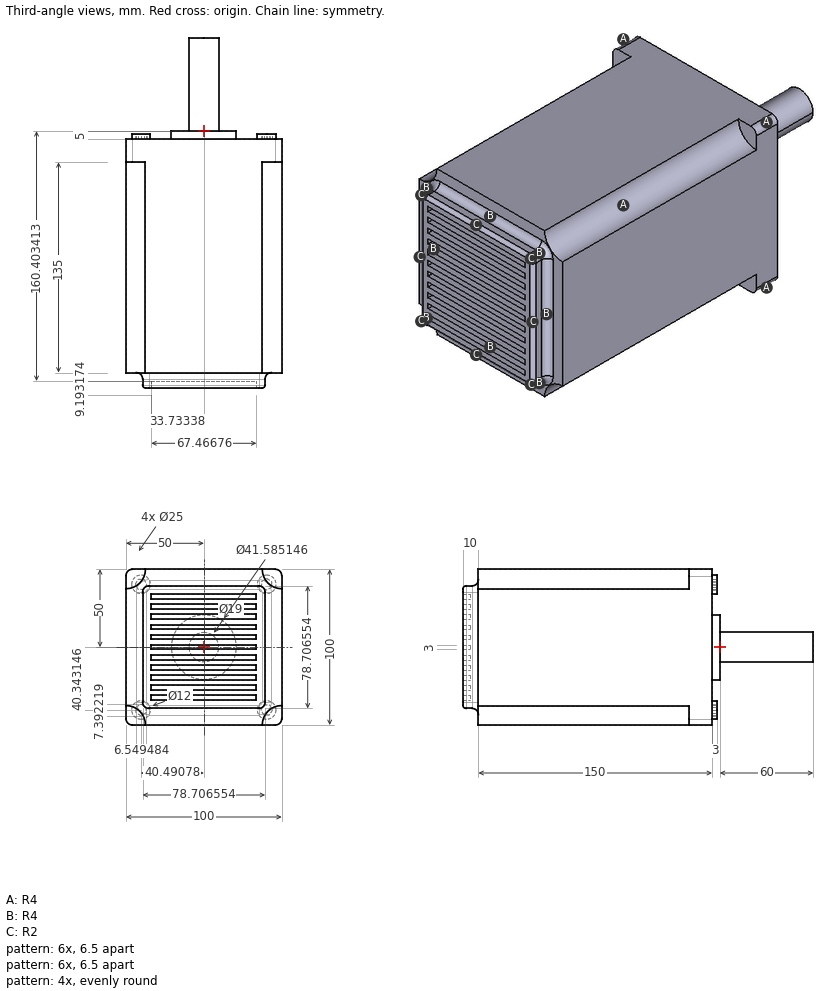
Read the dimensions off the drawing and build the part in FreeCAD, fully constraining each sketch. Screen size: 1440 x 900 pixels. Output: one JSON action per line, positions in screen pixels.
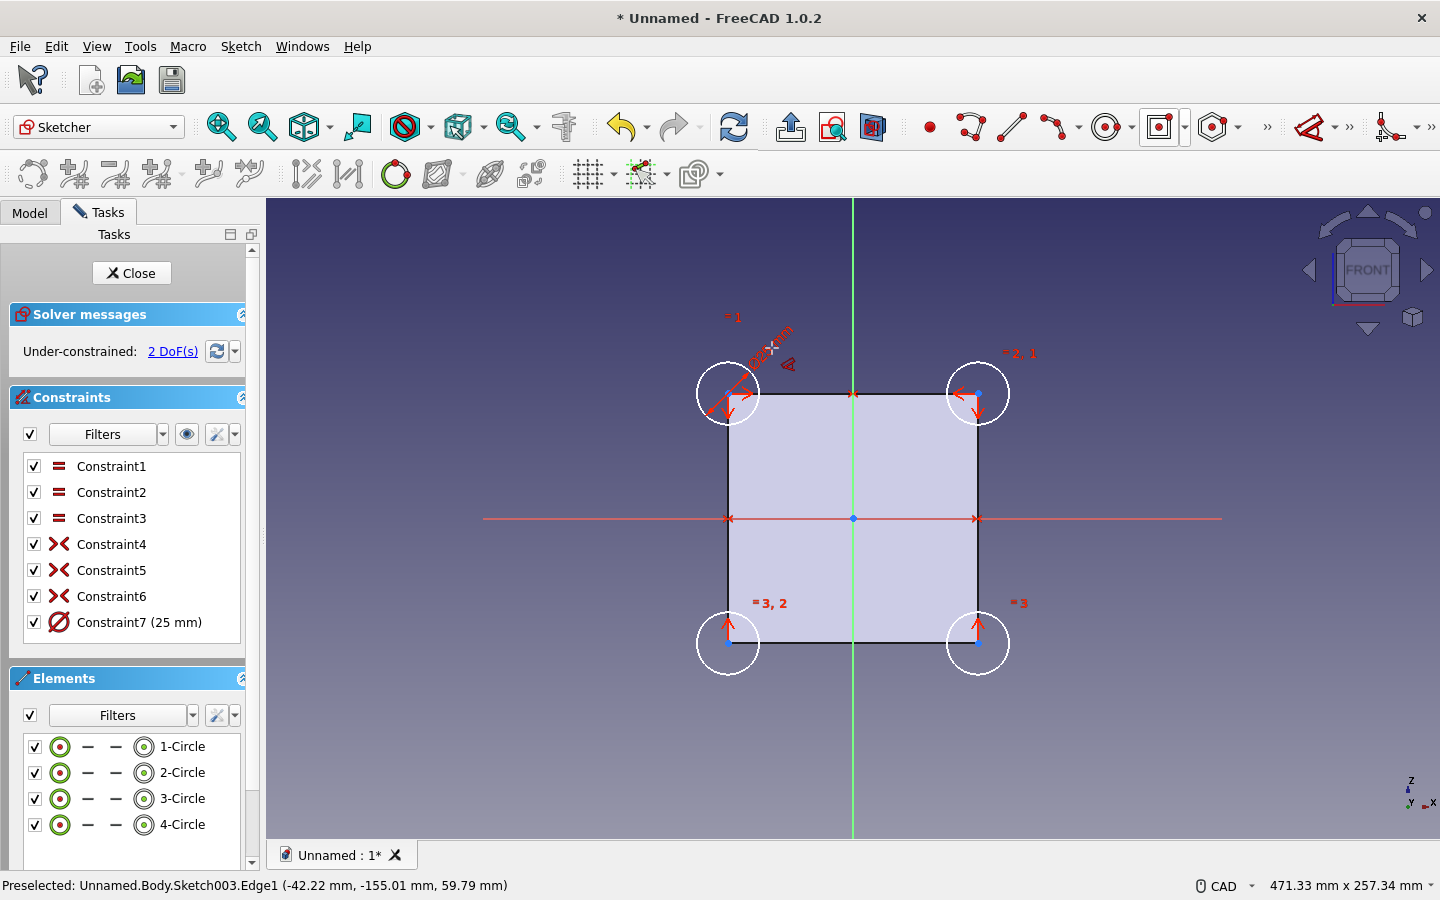
{"action": "left_click", "coordinate": [728, 394]}
{"action": "left_click", "coordinate": [791, 552]}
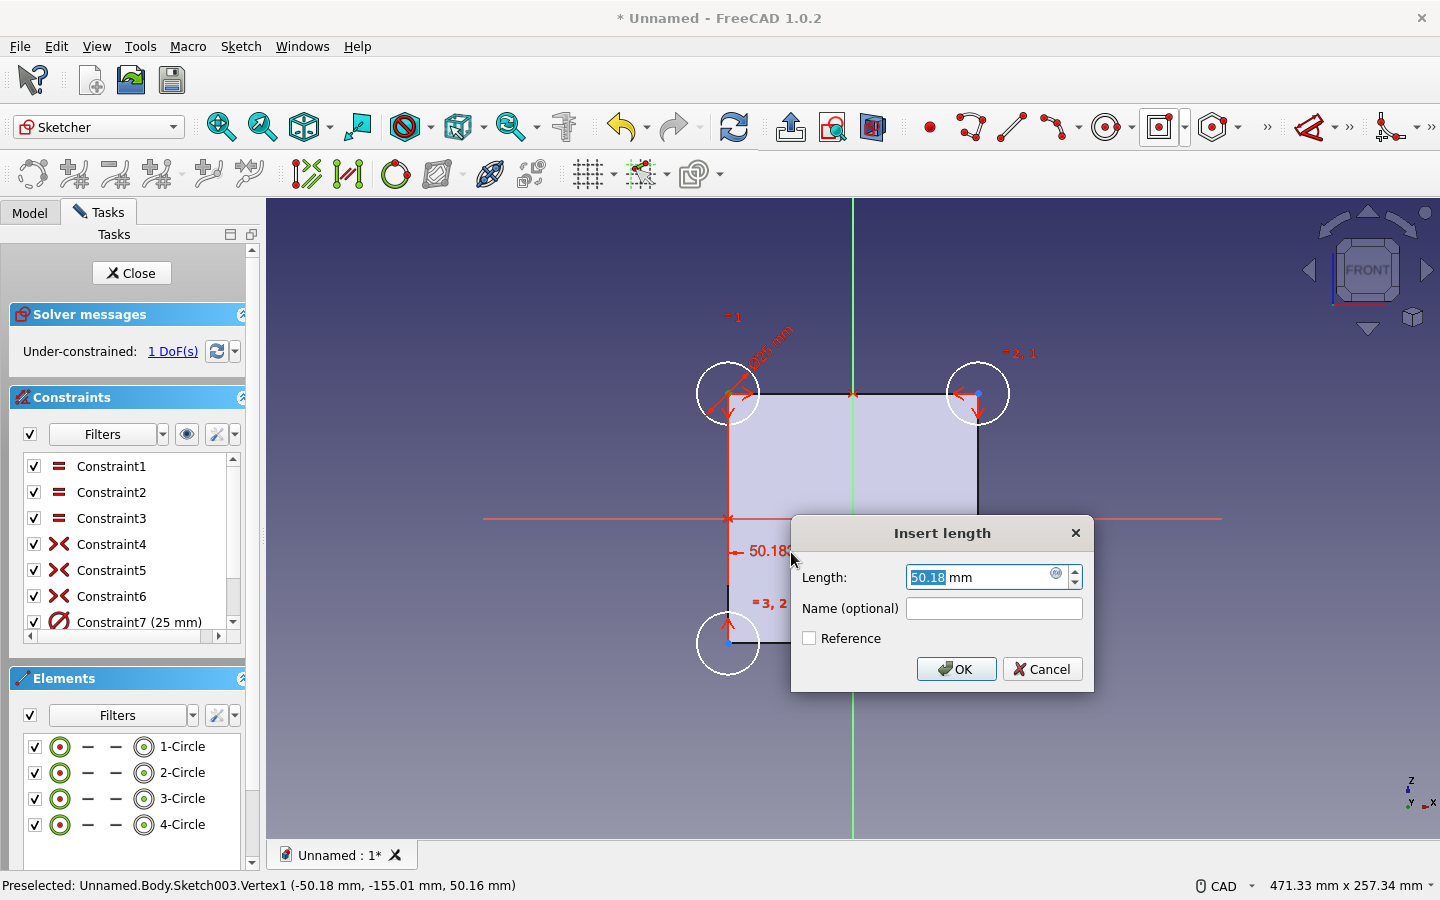
{"action": "type", "text": "50"}
{"action": "key", "text": "Return"}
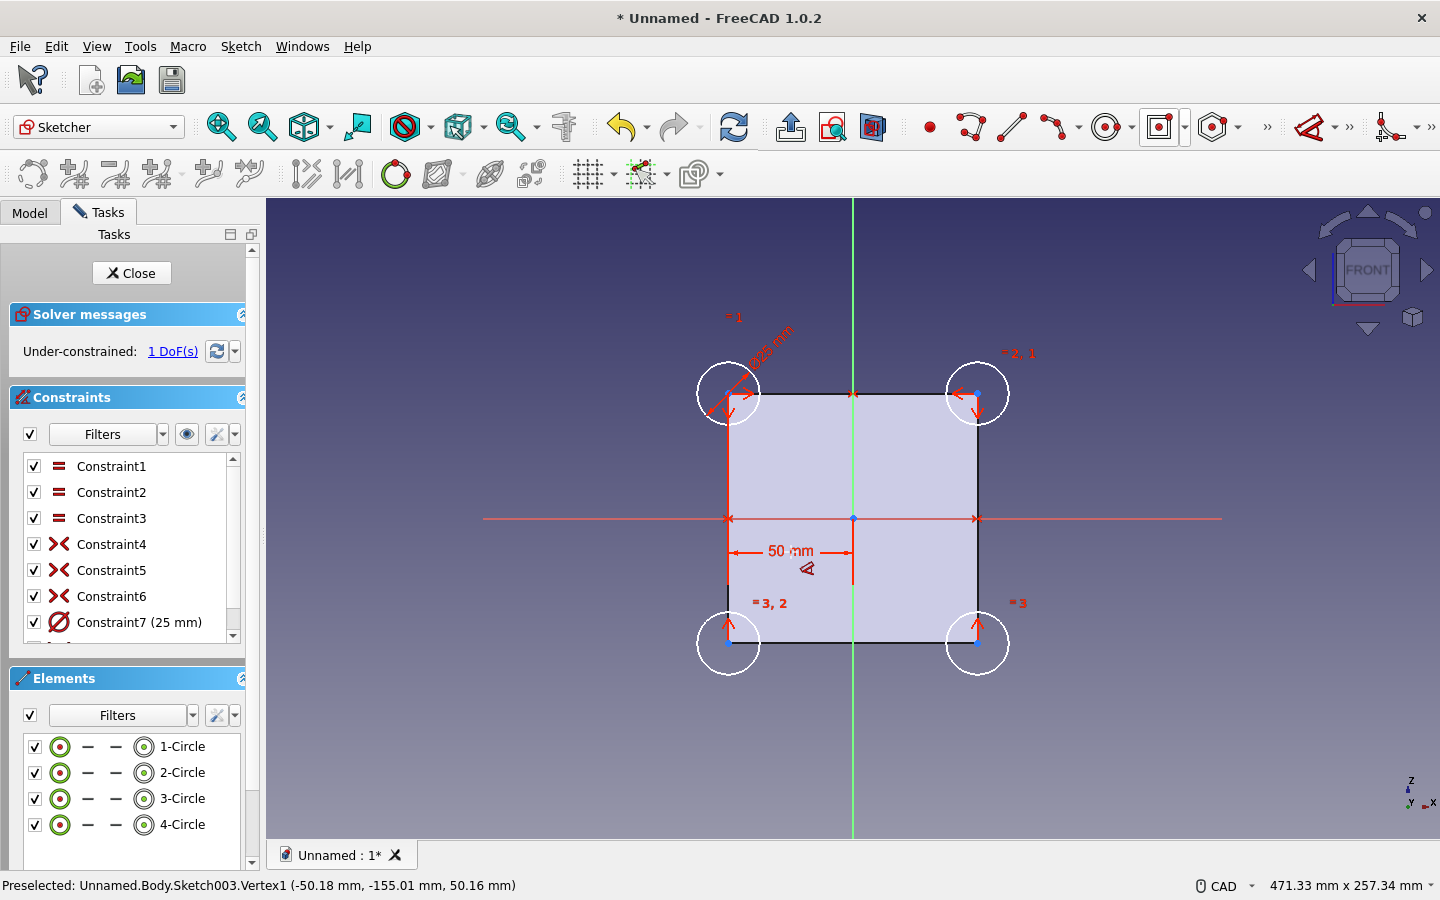
{"action": "left_click", "coordinate": [728, 394]}
{"action": "left_click", "coordinate": [694, 456]}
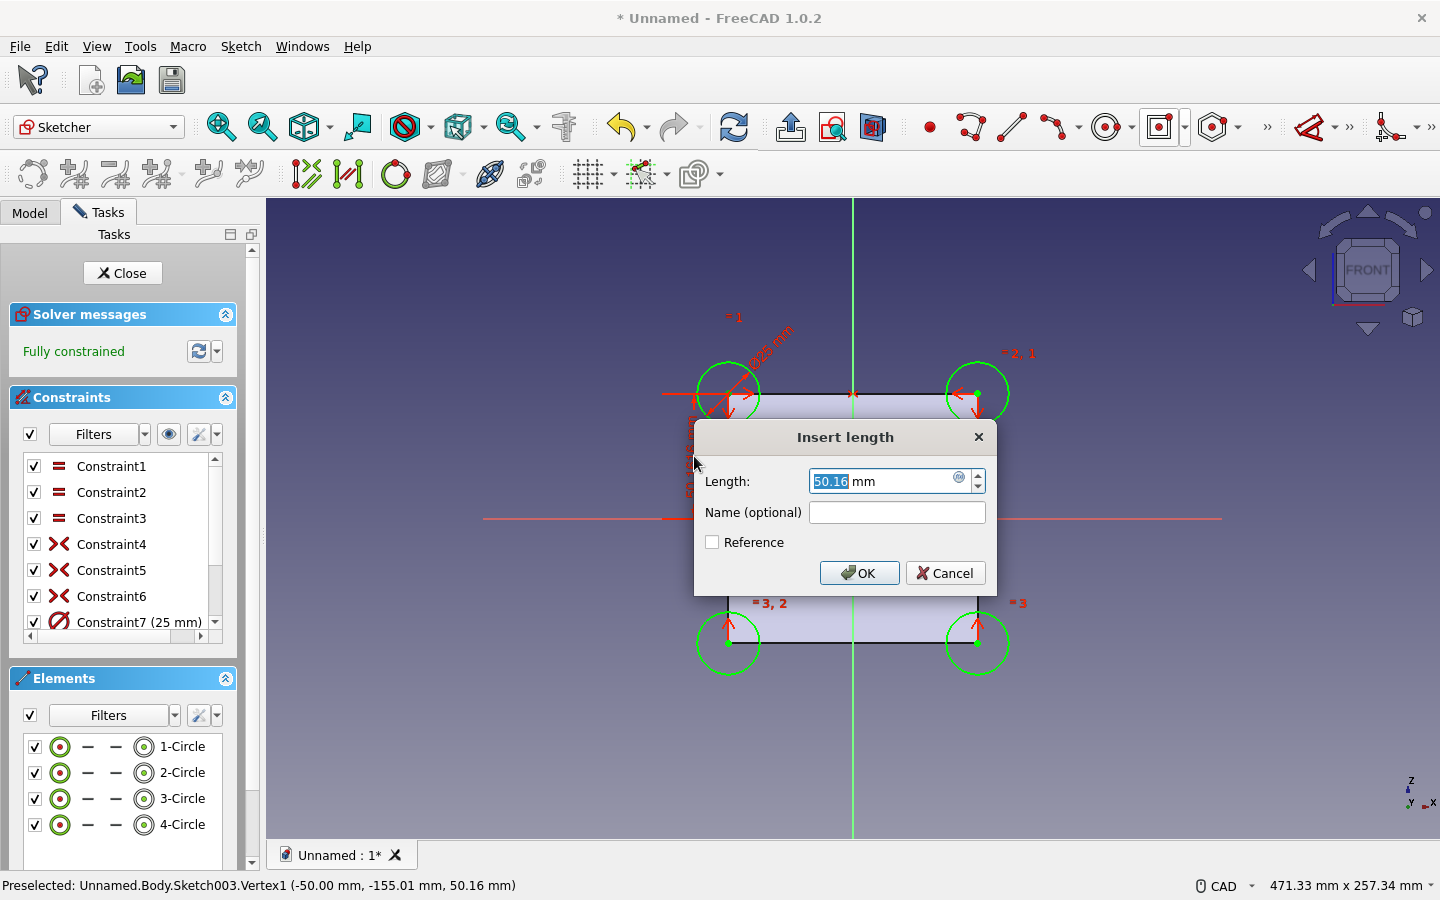
{"action": "type", "text": "50"}
{"action": "key", "text": "Return"}
{"action": "key", "text": "Escape"}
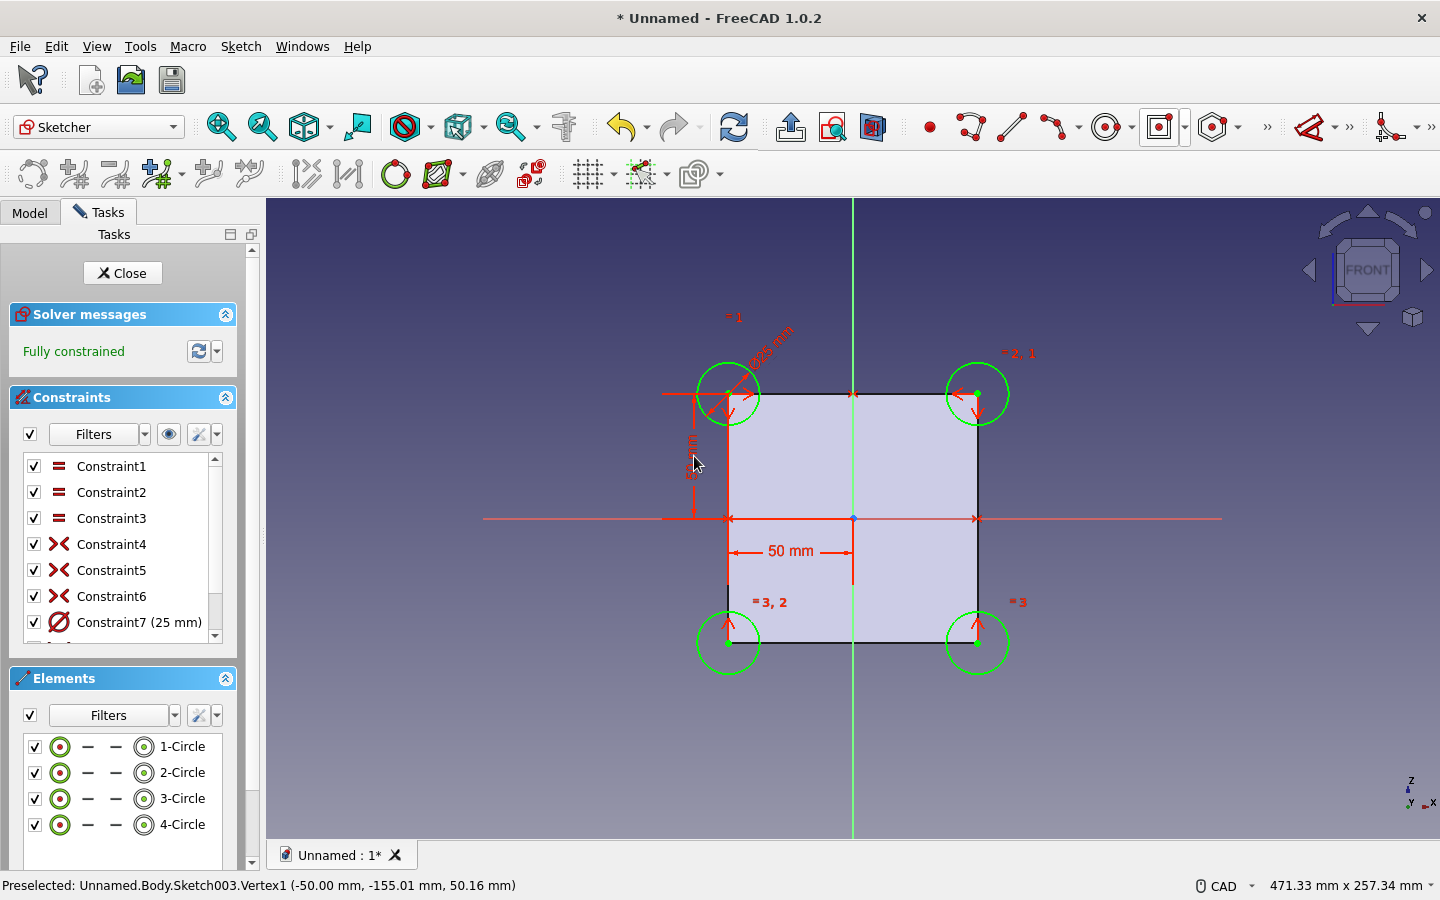
{"action": "left_click", "coordinate": [123, 273]}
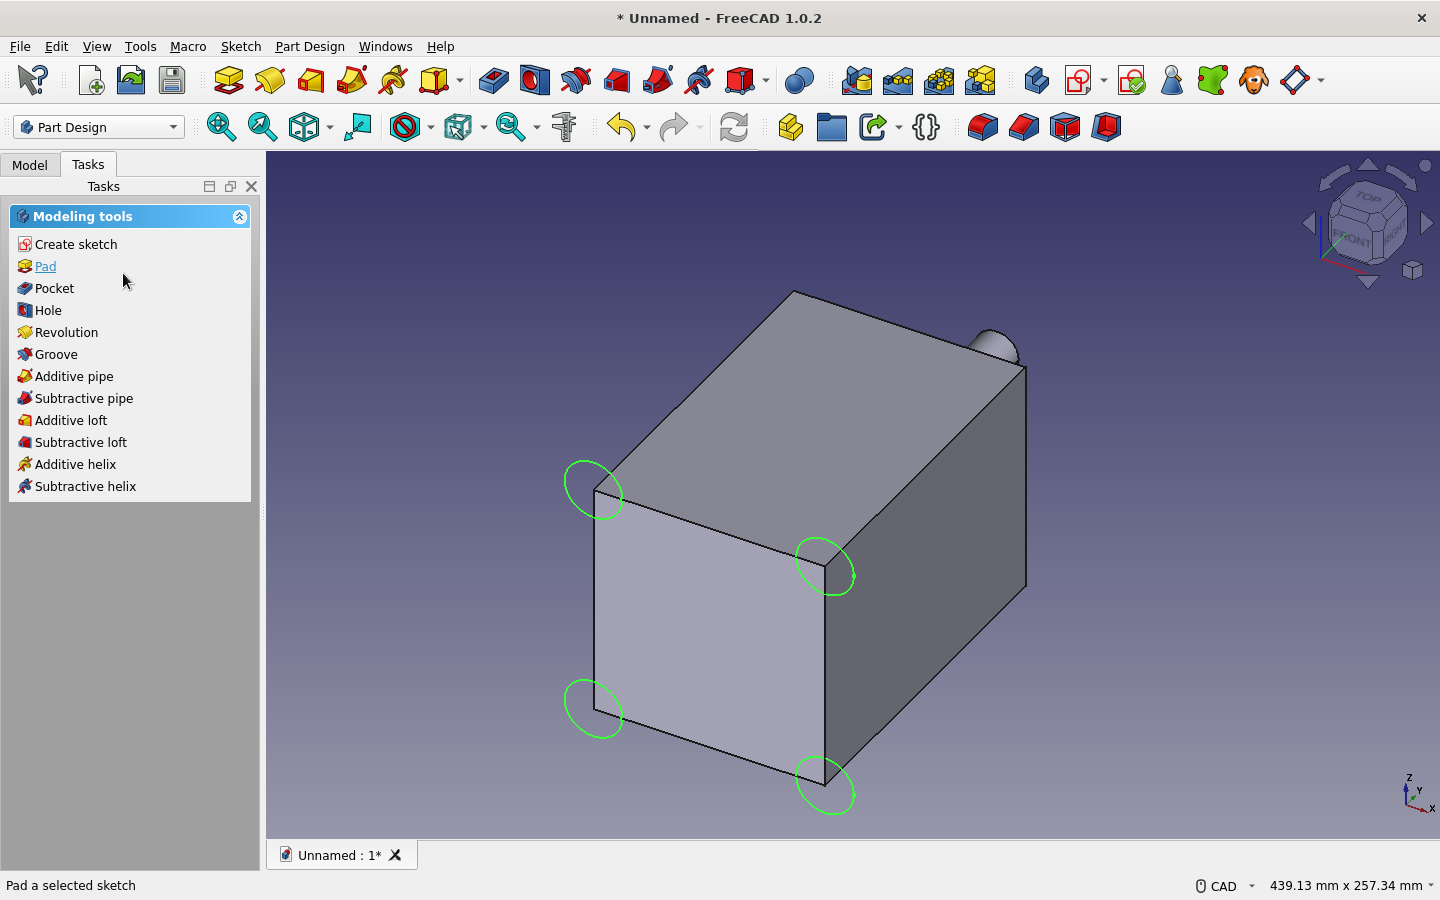
{"action": "left_click", "coordinate": [494, 80]}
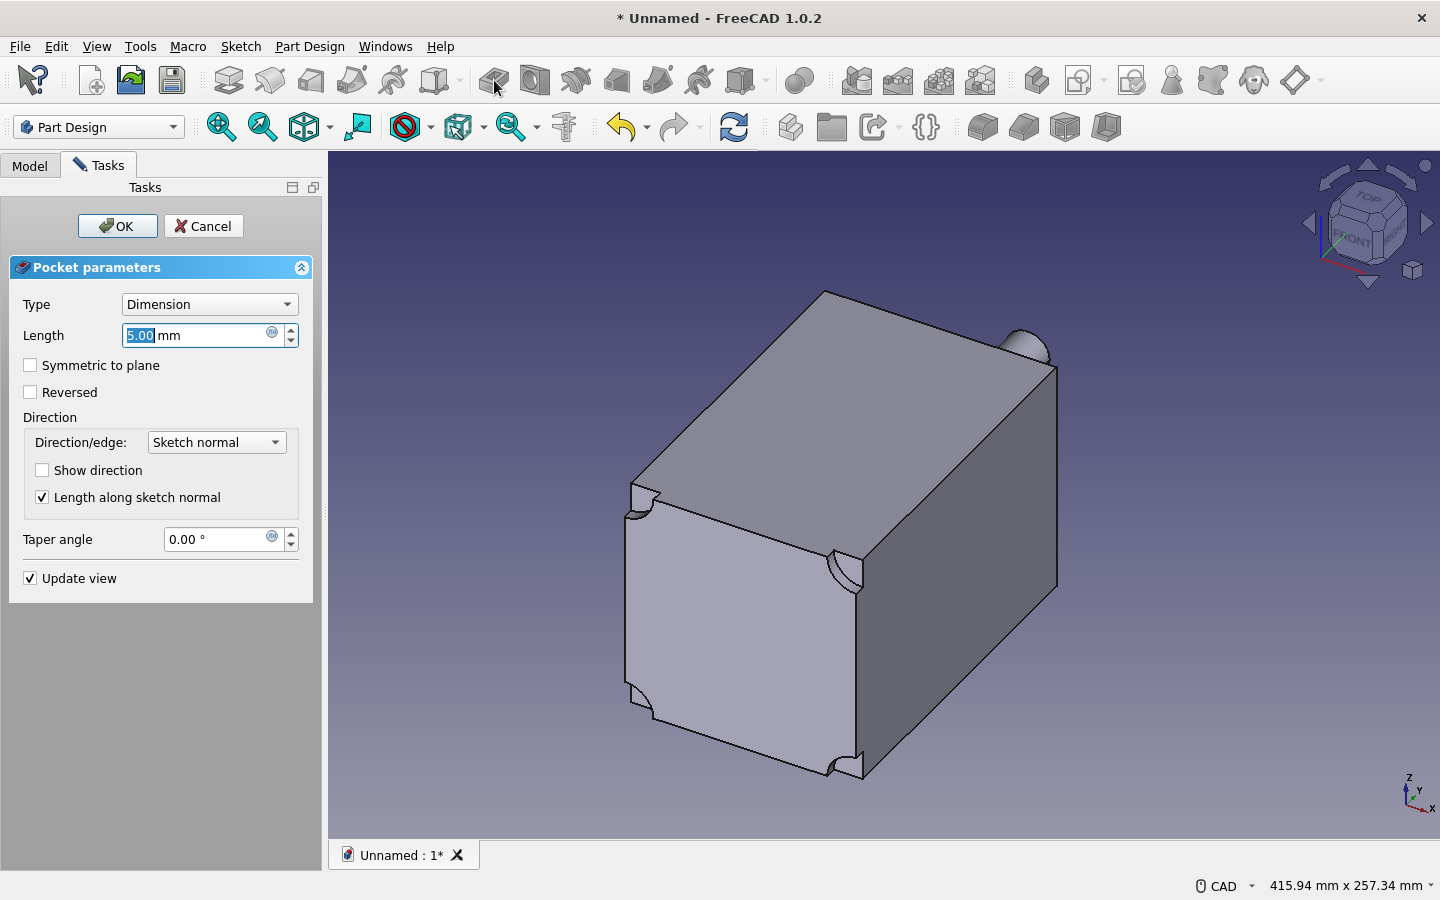
{"action": "type", "text": "135"}
{"action": "key", "text": "Tab"}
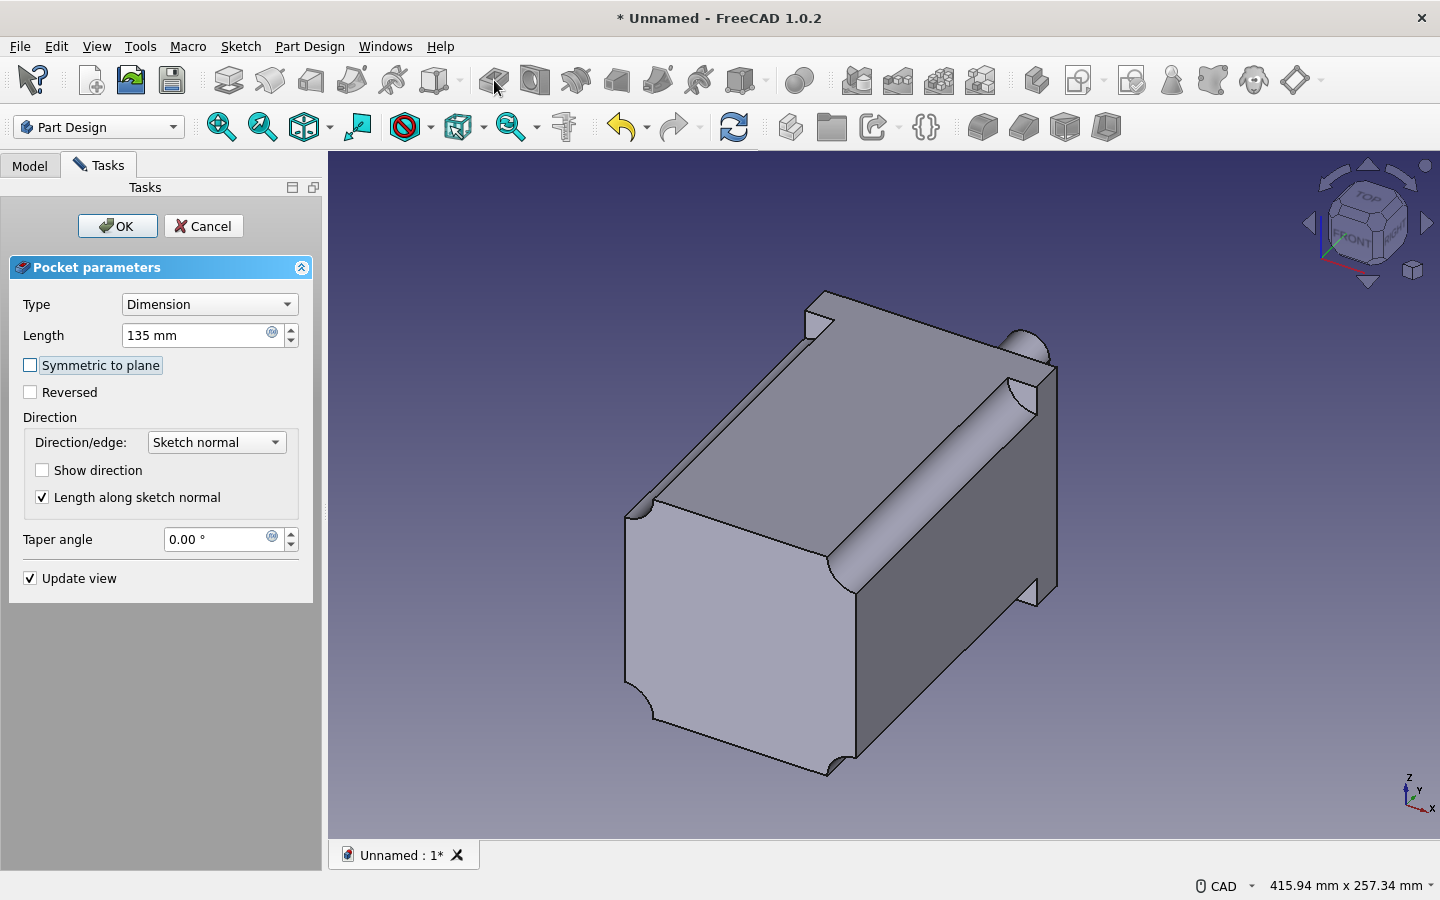
{"action": "left_click", "coordinate": [118, 226]}